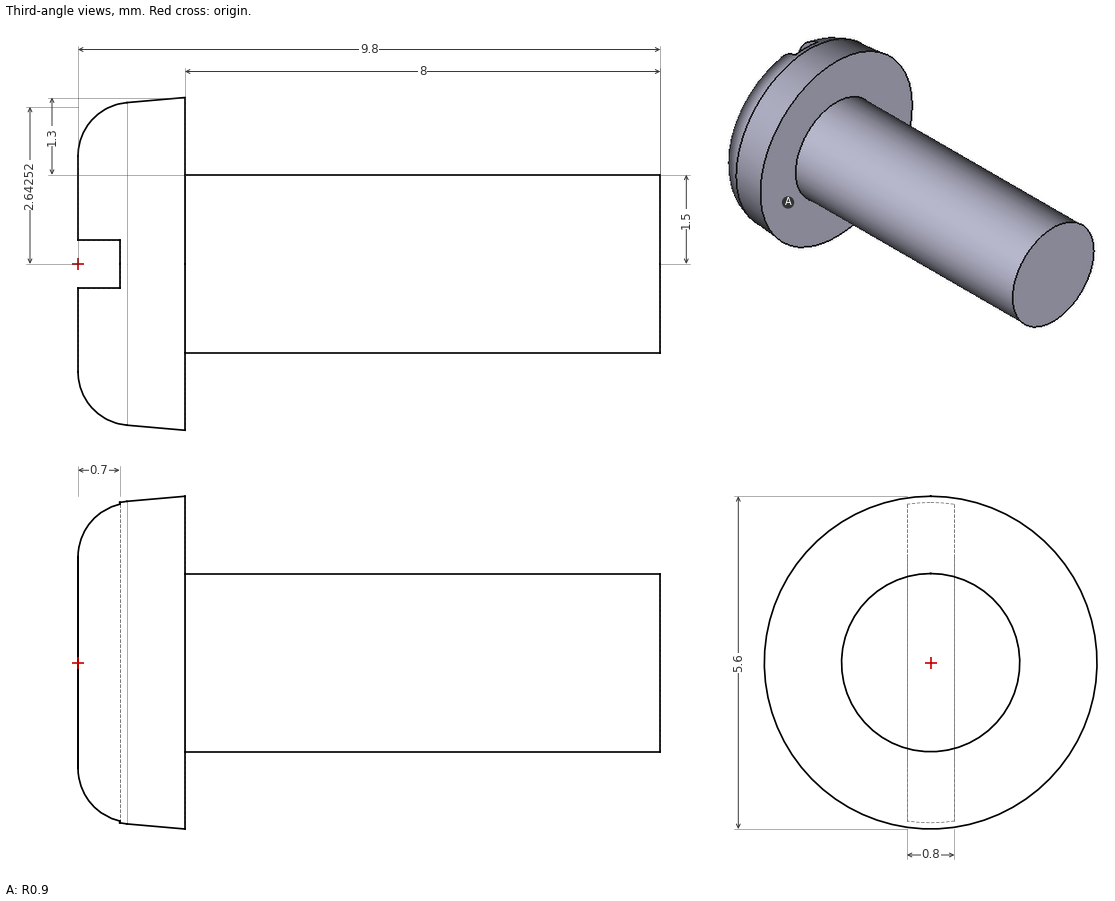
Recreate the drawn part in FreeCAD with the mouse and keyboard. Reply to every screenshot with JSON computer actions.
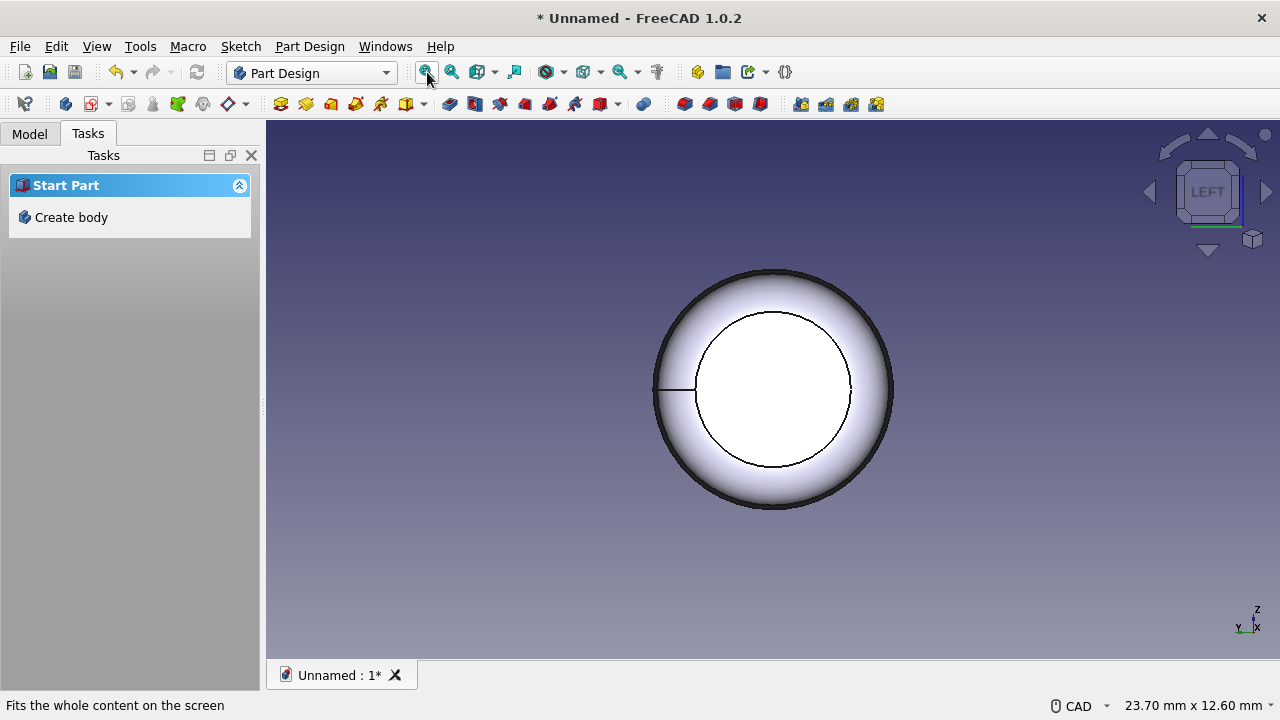
{"action": "left_click", "coordinate": [773, 388]}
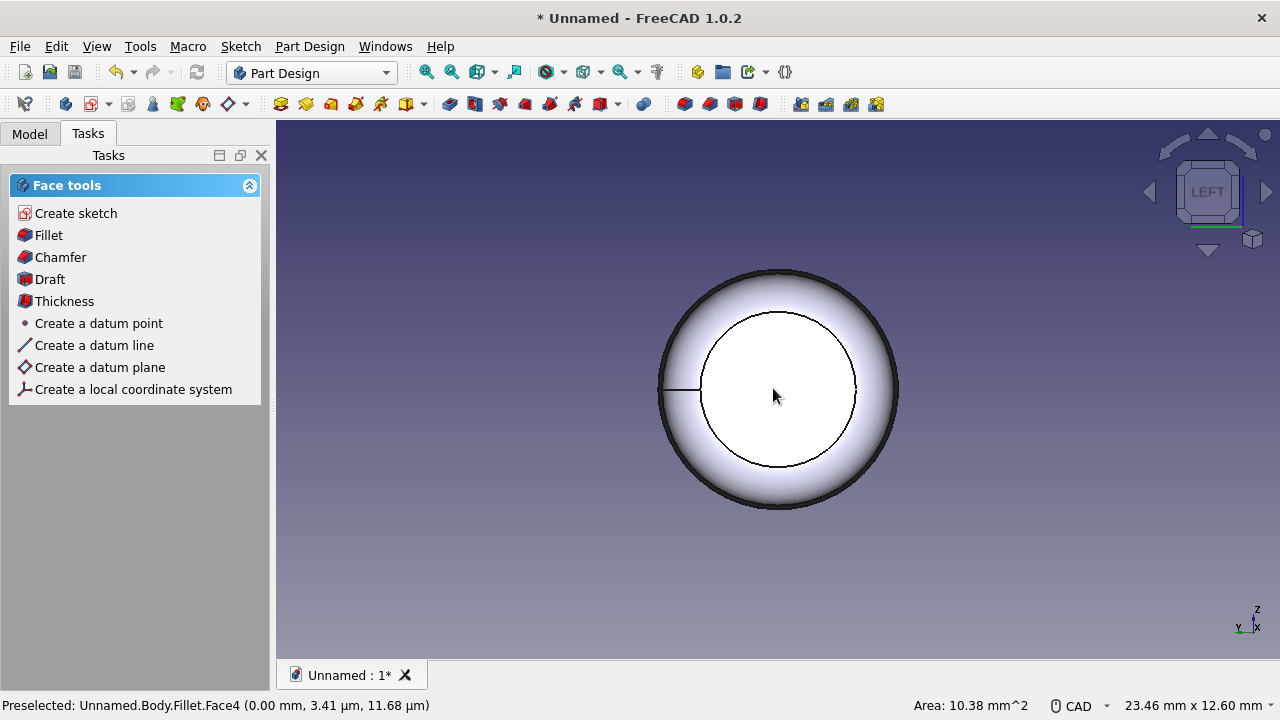
{"action": "left_click", "coordinate": [90, 104]}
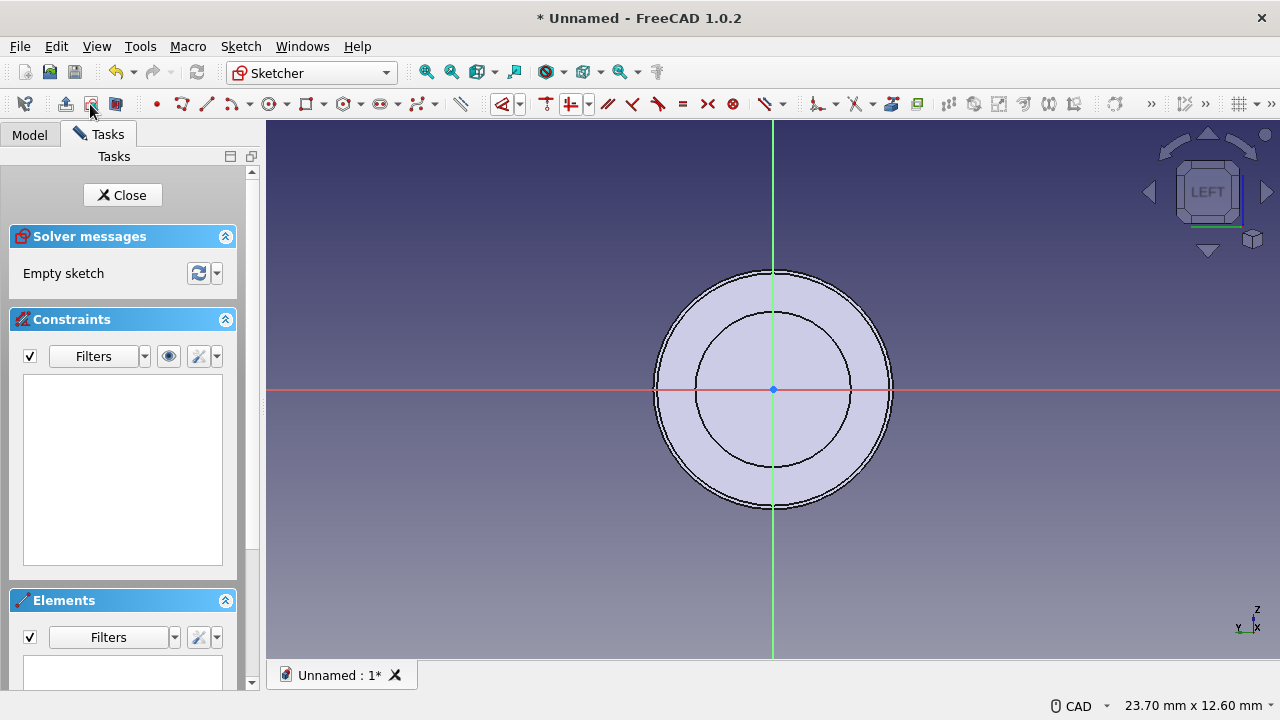
{"action": "scroll", "coordinate": [913, 390], "scroll_direction": "up", "scroll_amount": 2}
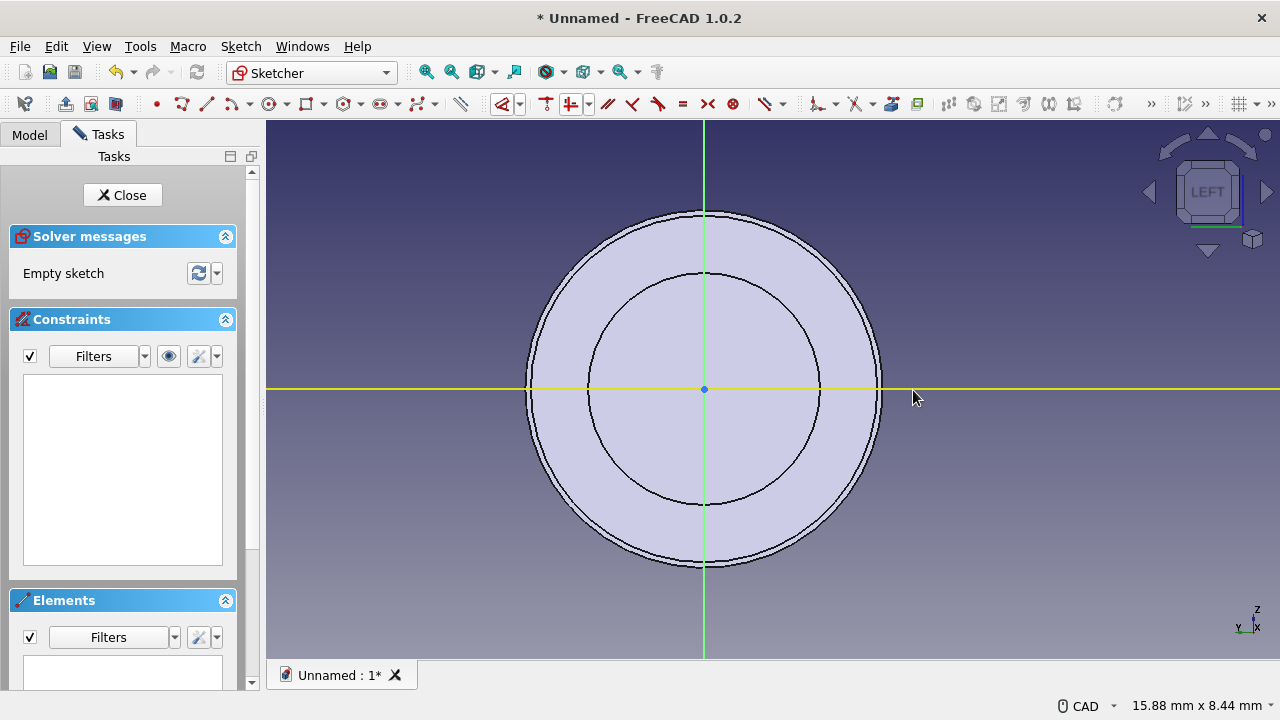
{"action": "left_click", "coordinate": [324, 104]}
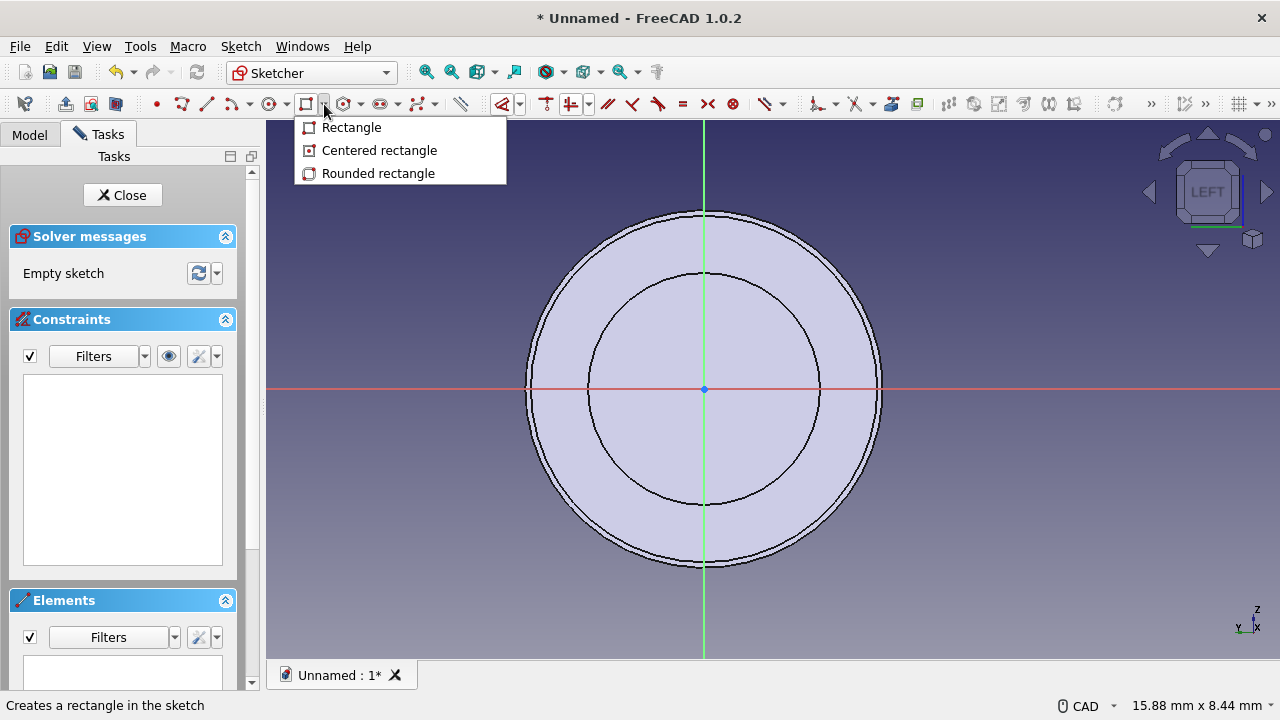
{"action": "left_click", "coordinate": [400, 150]}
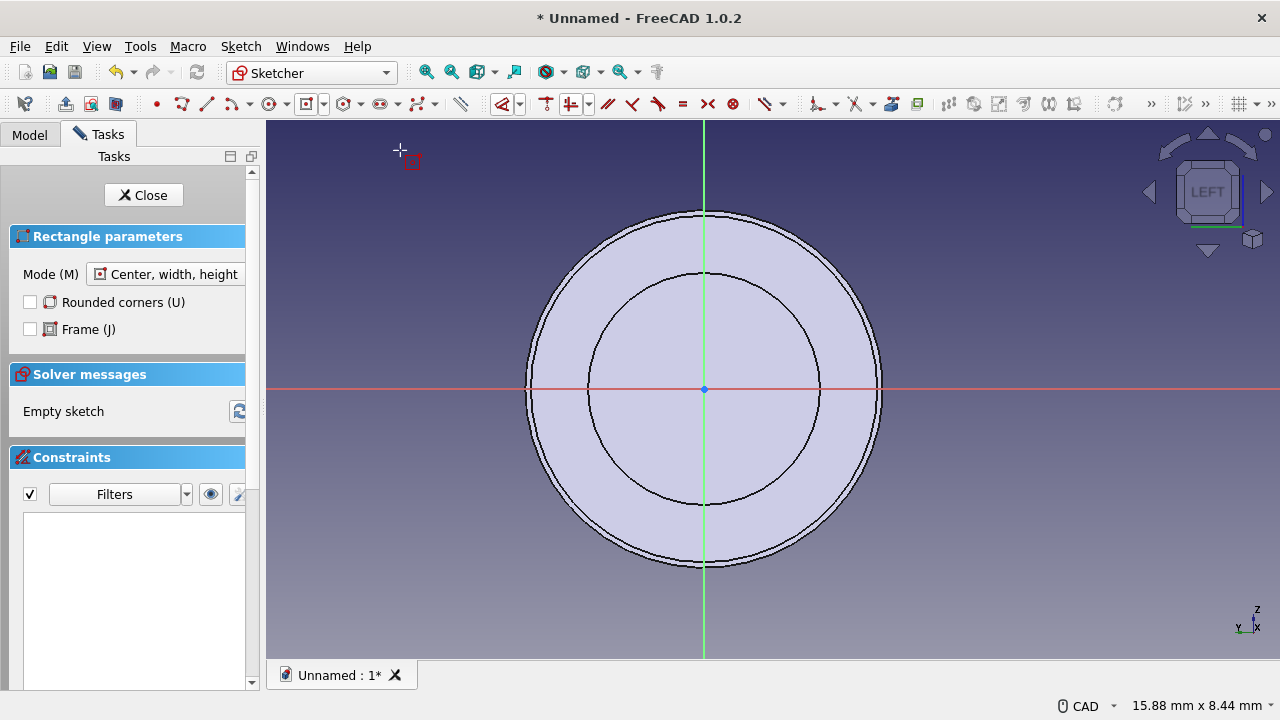
{"action": "left_click", "coordinate": [704, 389]}
{"action": "left_click", "coordinate": [730, 210]}
{"action": "key", "text": "Escape"}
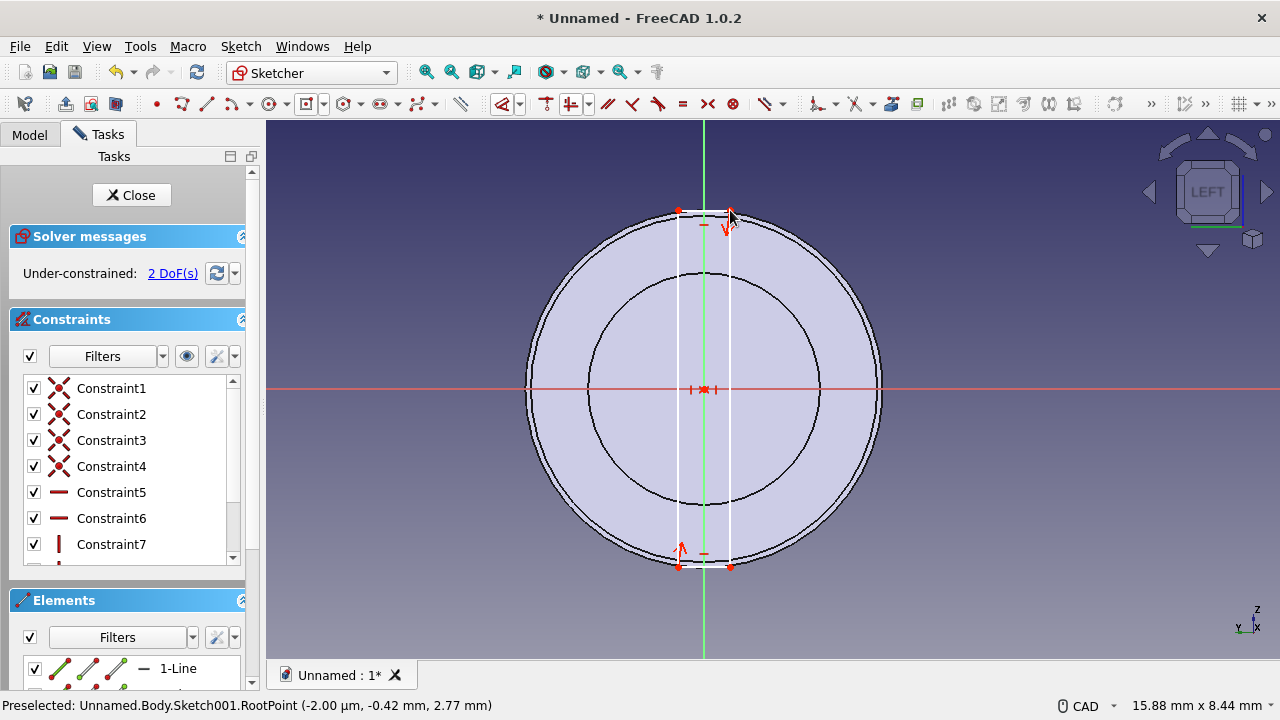
{"action": "scroll", "coordinate": [694, 567], "scroll_direction": "up", "scroll_amount": 2}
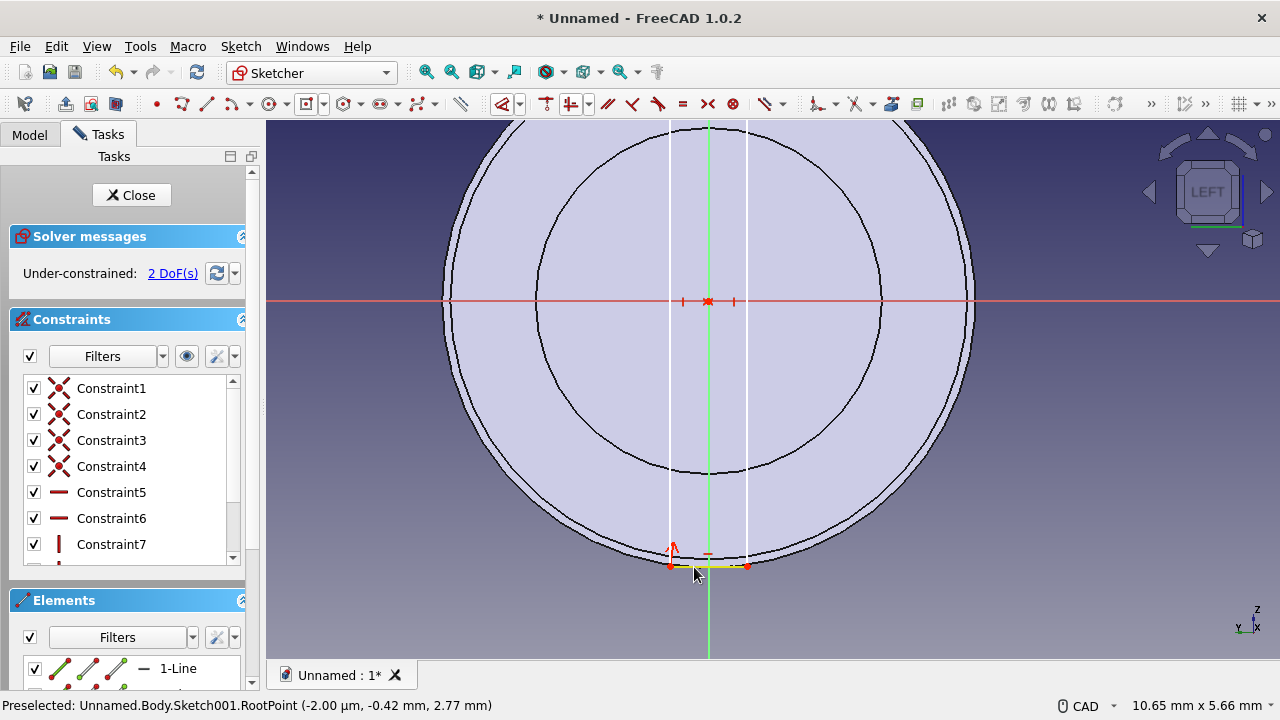
{"action": "left_click", "coordinate": [693, 567]}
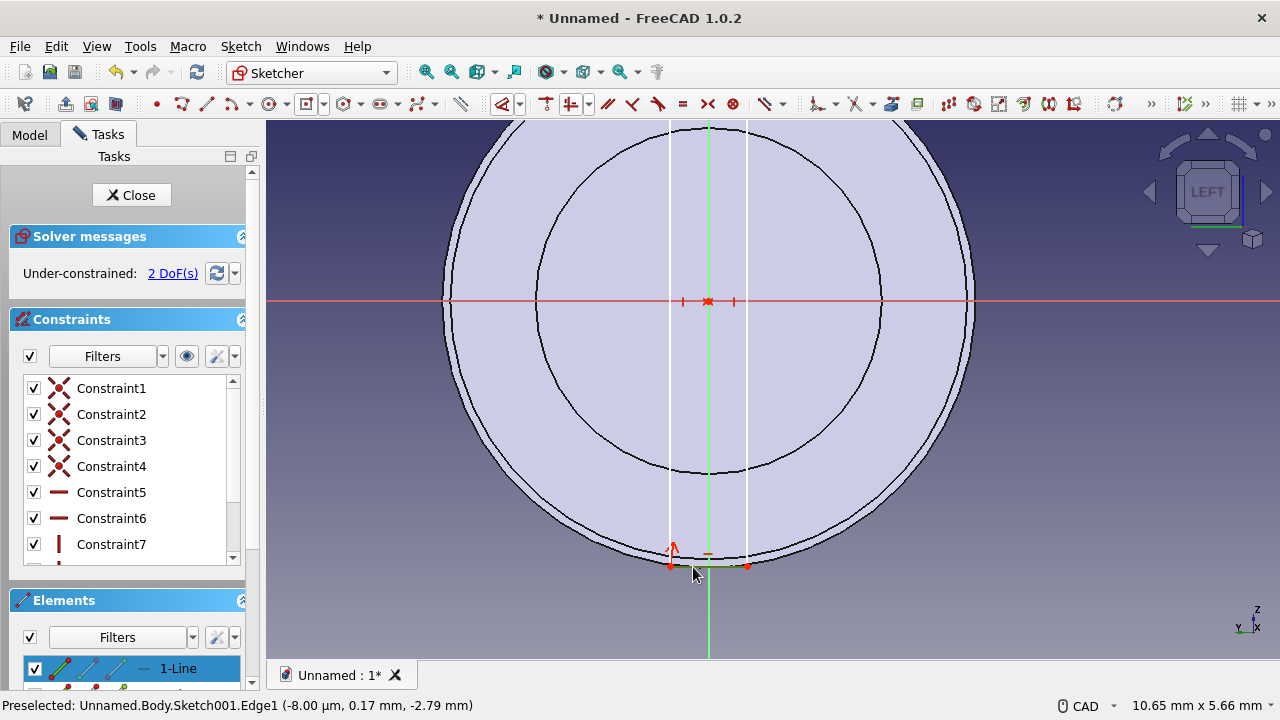
{"action": "left_click", "coordinate": [520, 104]}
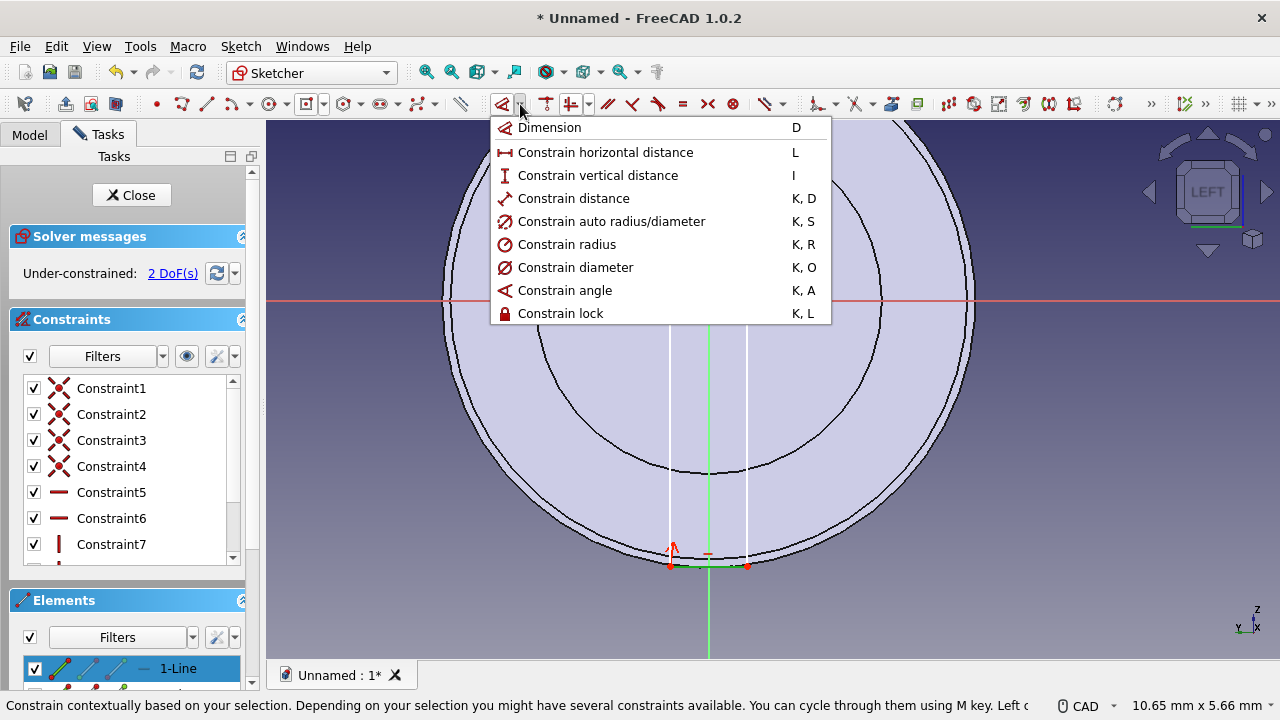
{"action": "left_click", "coordinate": [661, 152]}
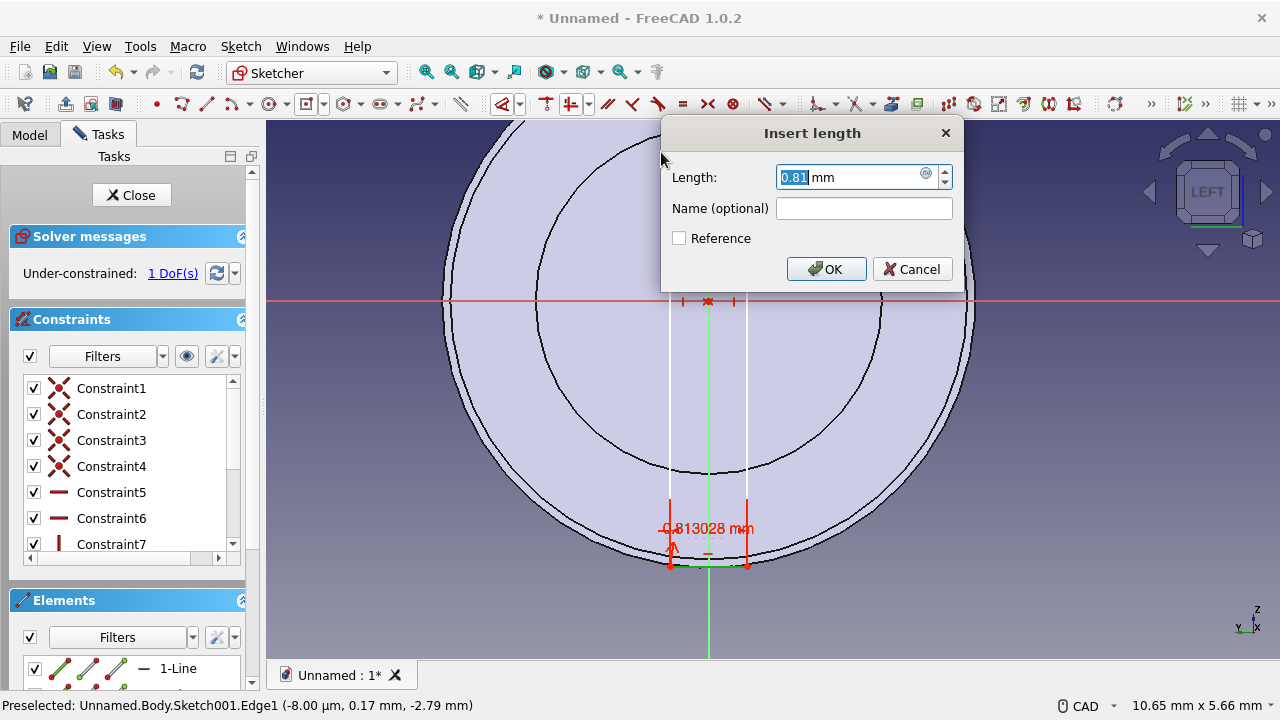
{"action": "type", "text": "0.8"}
{"action": "key", "text": "Return"}